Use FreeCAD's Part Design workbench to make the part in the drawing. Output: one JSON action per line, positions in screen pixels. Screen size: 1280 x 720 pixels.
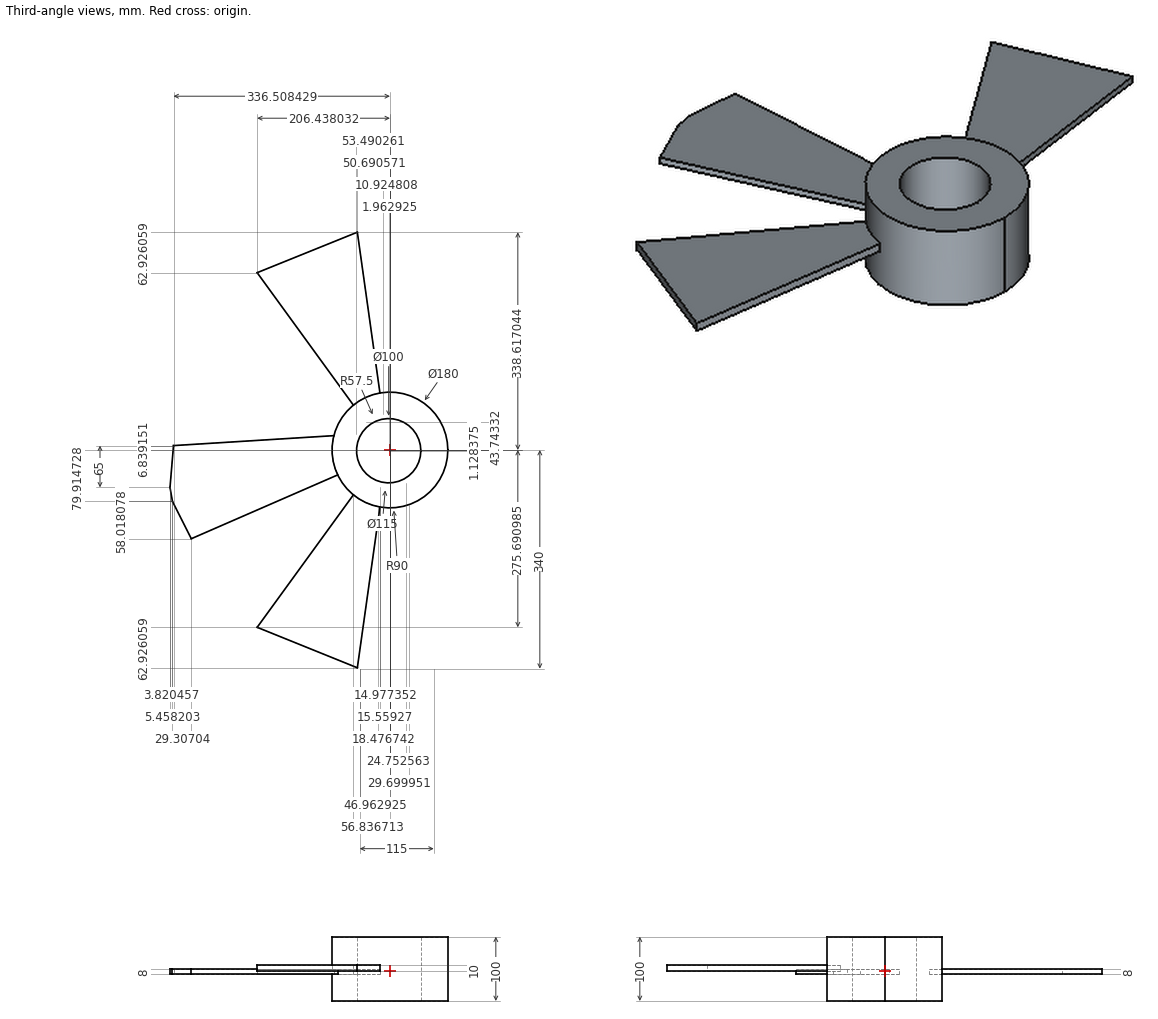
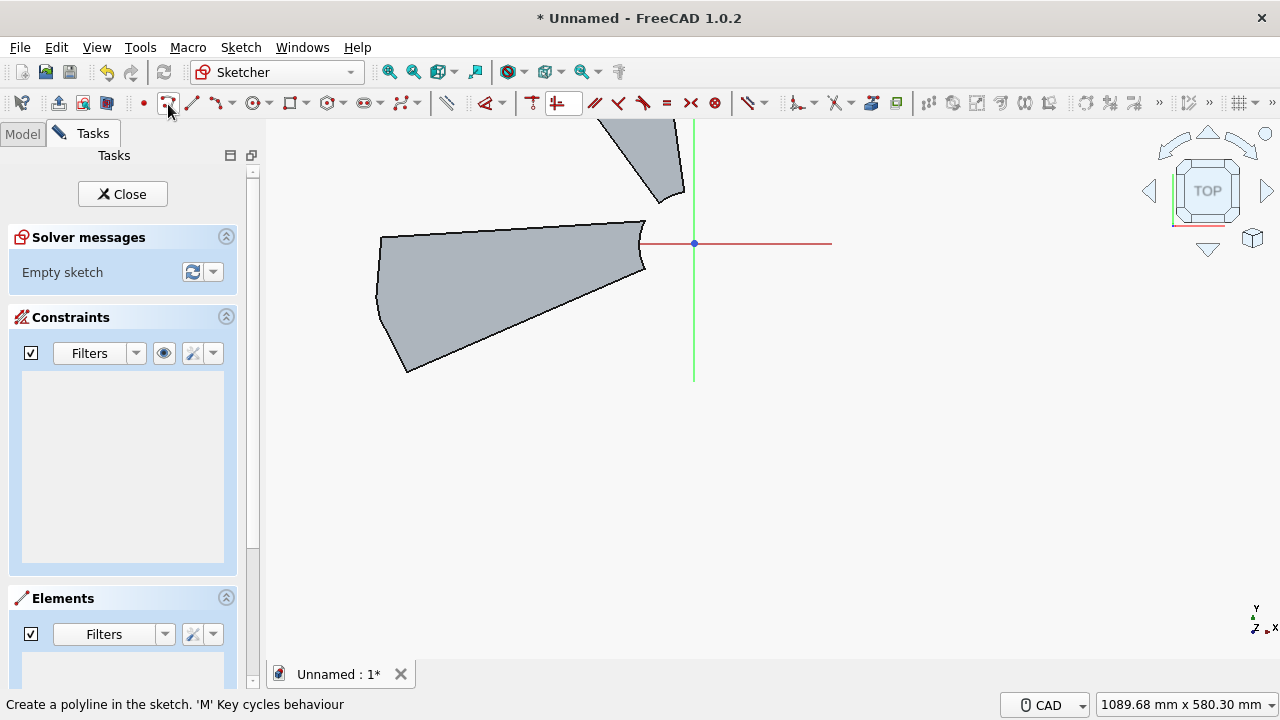
{"action": "left_click", "coordinate": [681, 297]}
{"action": "left_click", "coordinate": [651, 560]}
{"action": "left_click", "coordinate": [758, 560]}
{"action": "left_click", "coordinate": [718, 292]}
{"action": "right_click", "coordinate": [718, 292]}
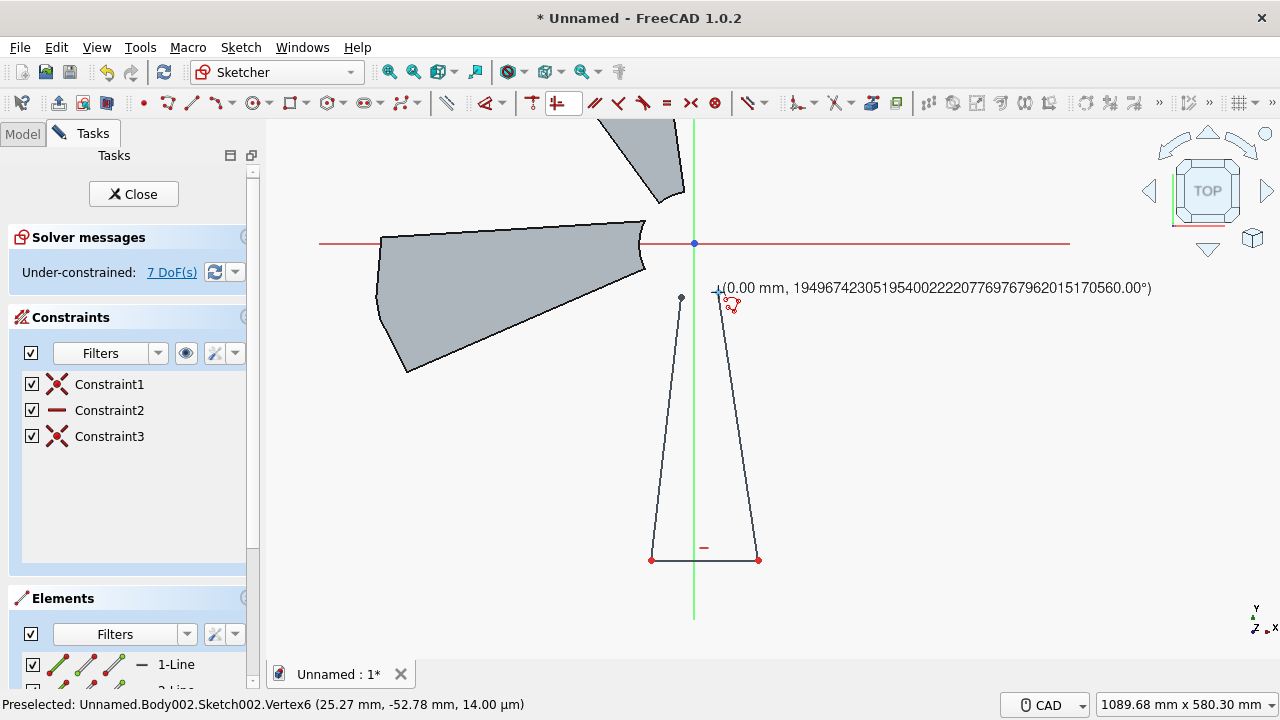
{"action": "left_click", "coordinate": [216, 104]}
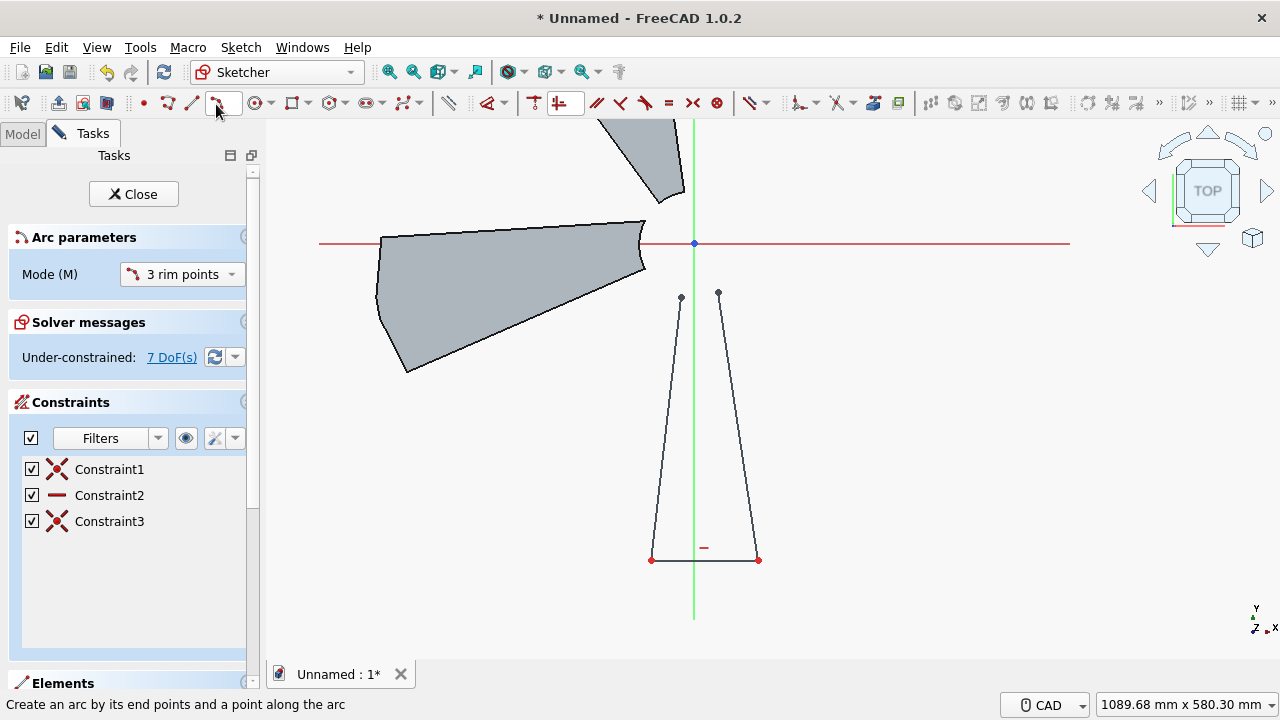
{"action": "left_click", "coordinate": [718, 293]}
{"action": "left_click", "coordinate": [681, 298]}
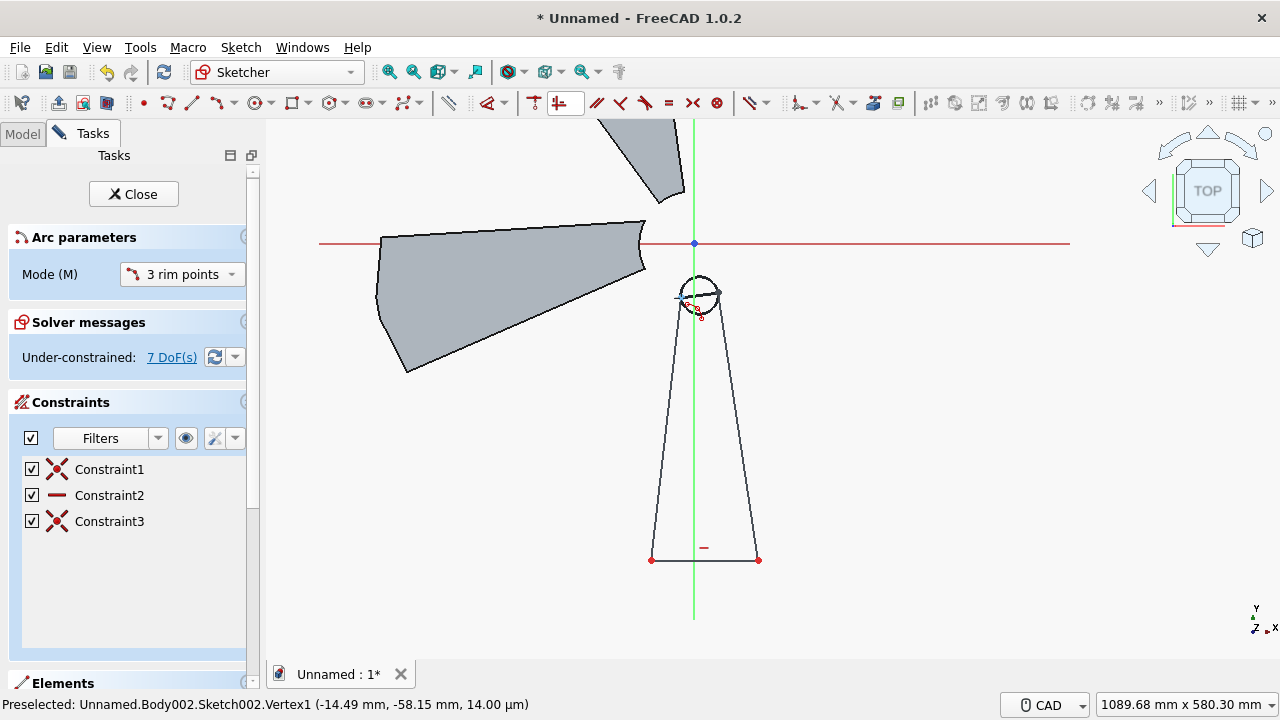
{"action": "scroll", "coordinate": [699, 298], "scroll_direction": "up", "scroll_amount": 8}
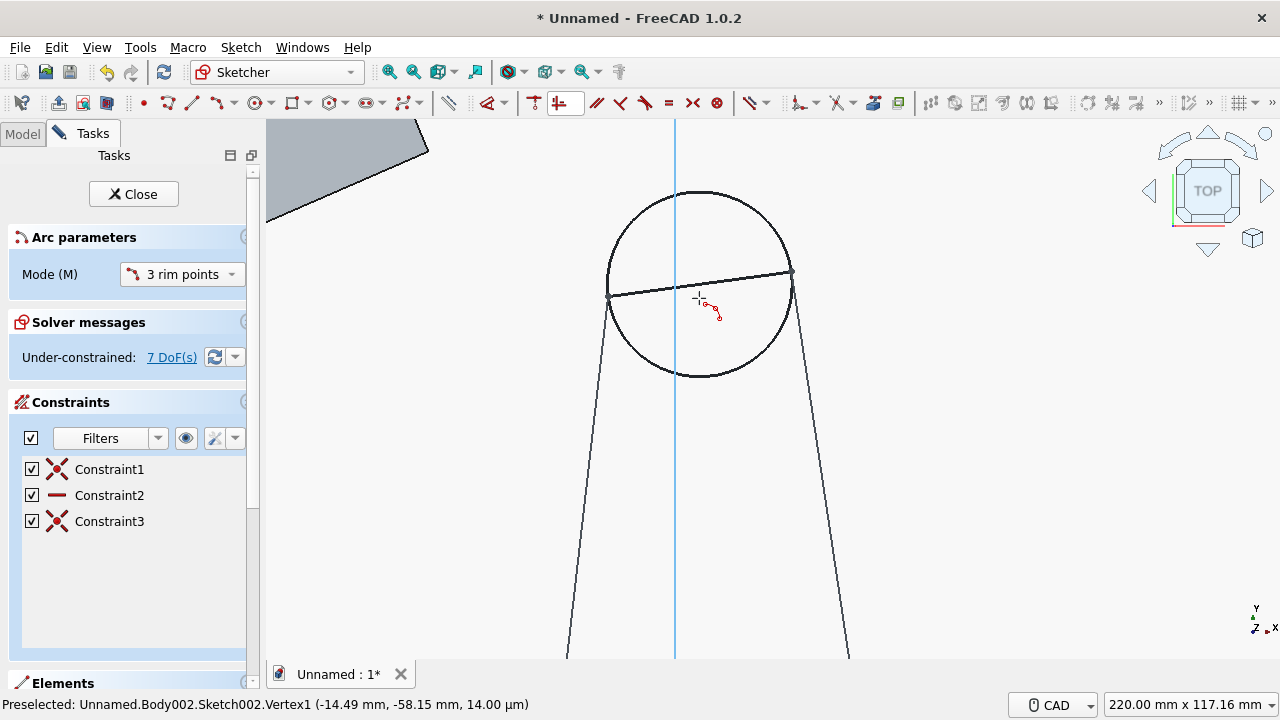
{"action": "left_click", "coordinate": [700, 297]}
{"action": "key", "text": "Escape"}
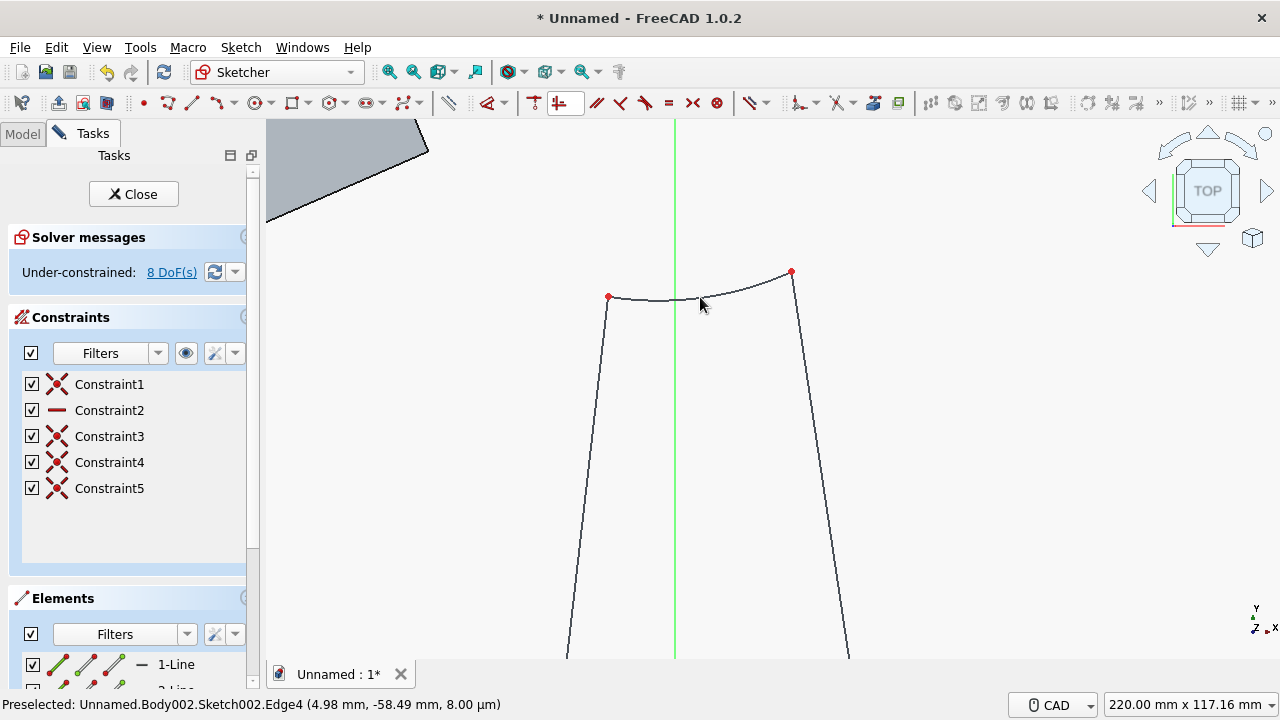
{"action": "left_click", "coordinate": [488, 104]}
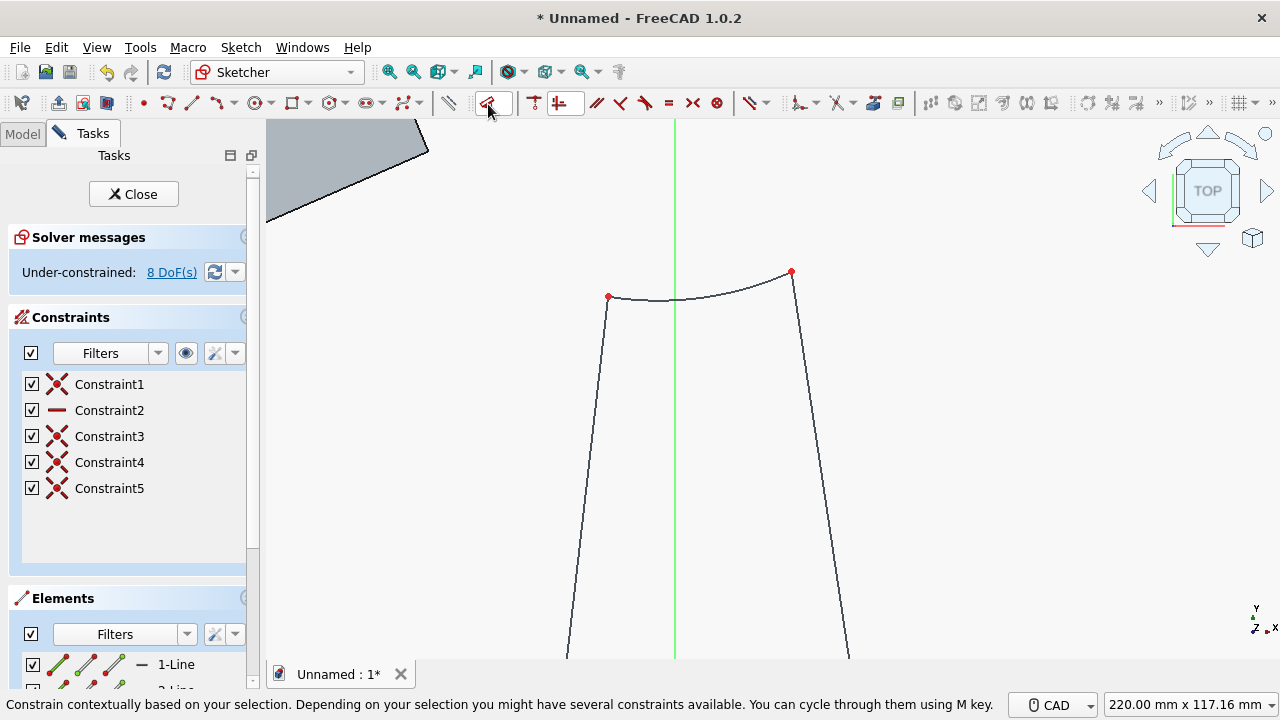
{"action": "scroll", "coordinate": [664, 301], "scroll_direction": "up", "scroll_amount": 2}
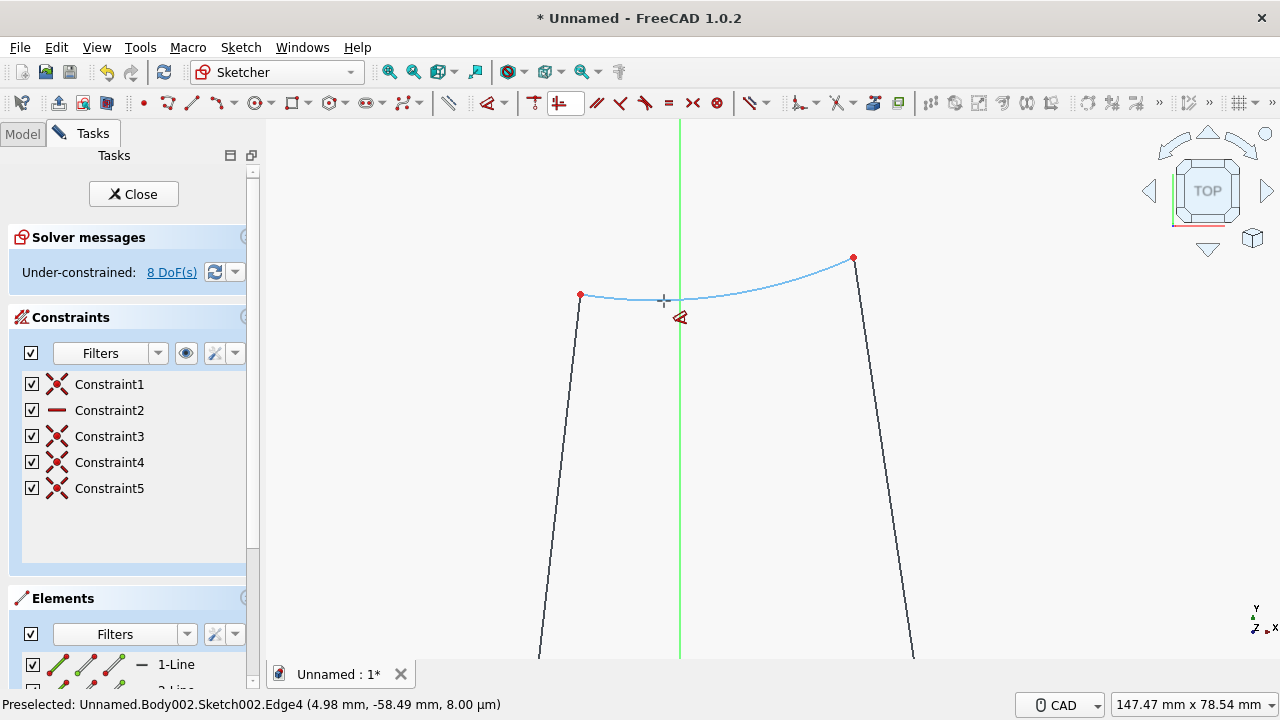
{"action": "left_click", "coordinate": [664, 300]}
{"action": "left_click", "coordinate": [665, 332]}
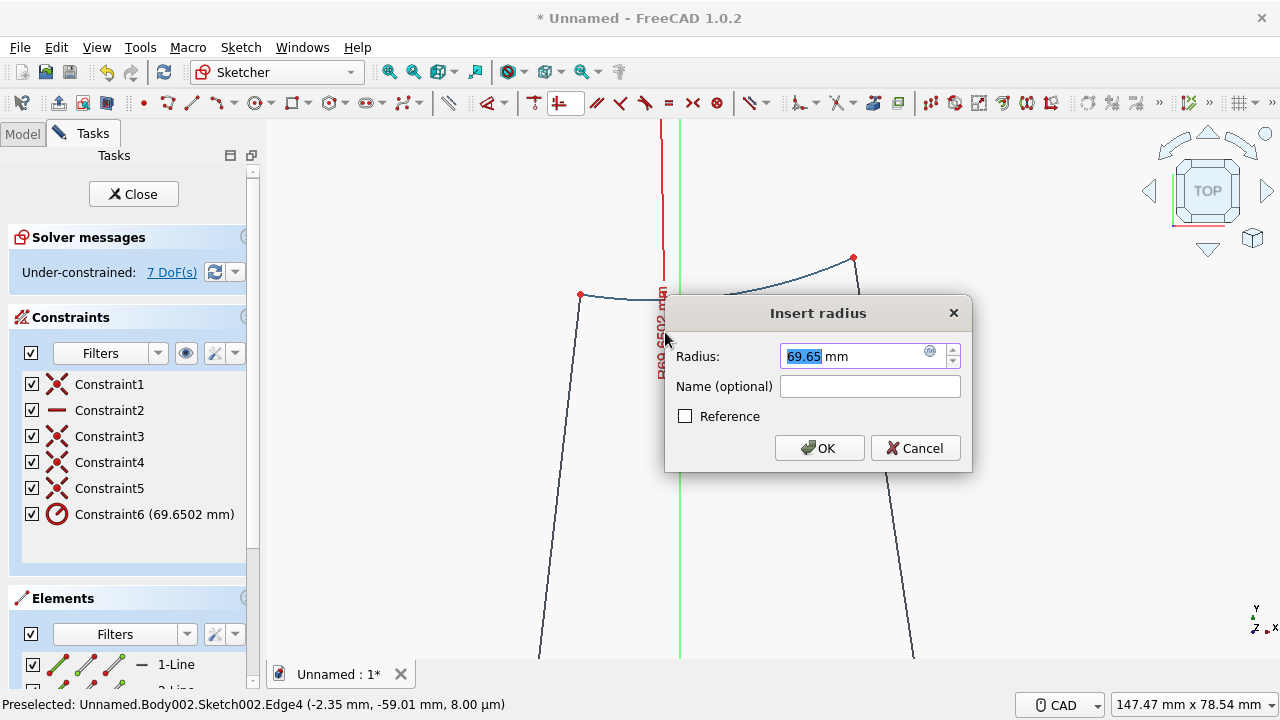
{"action": "type", "text": "57.5"}
{"action": "key", "text": "Return"}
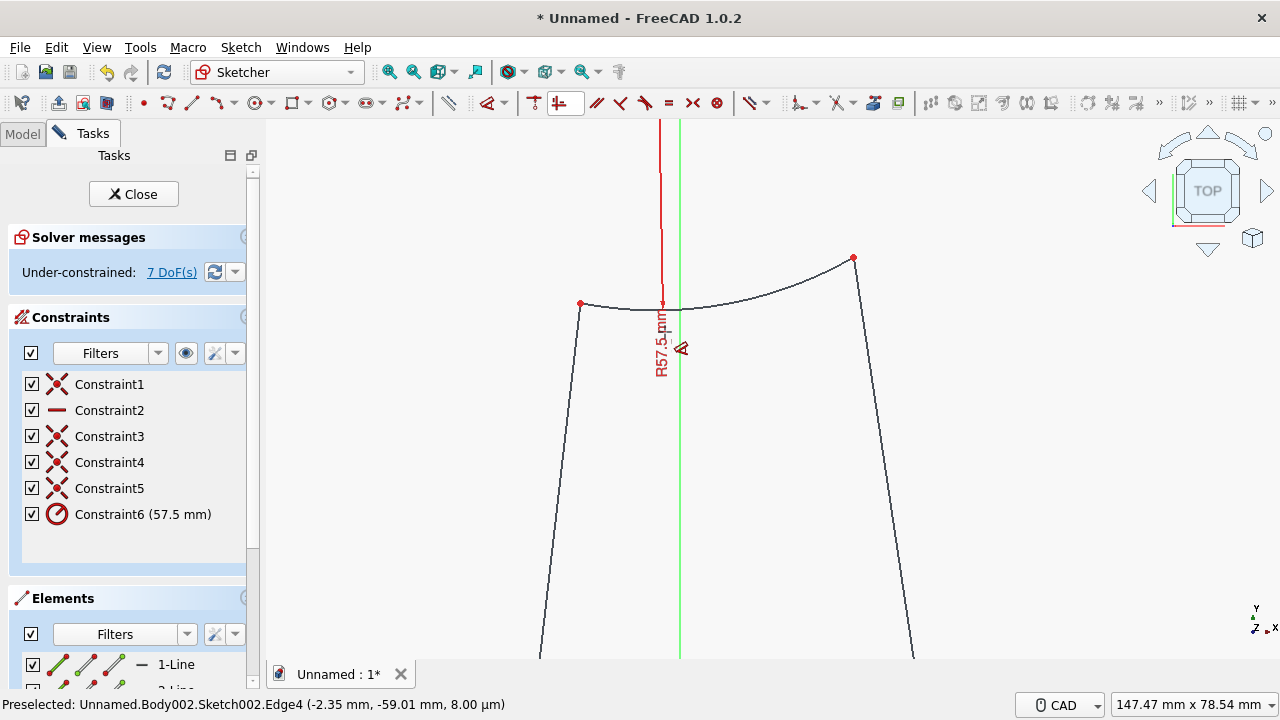
{"action": "scroll", "coordinate": [697, 283], "scroll_direction": "down", "scroll_amount": 10}